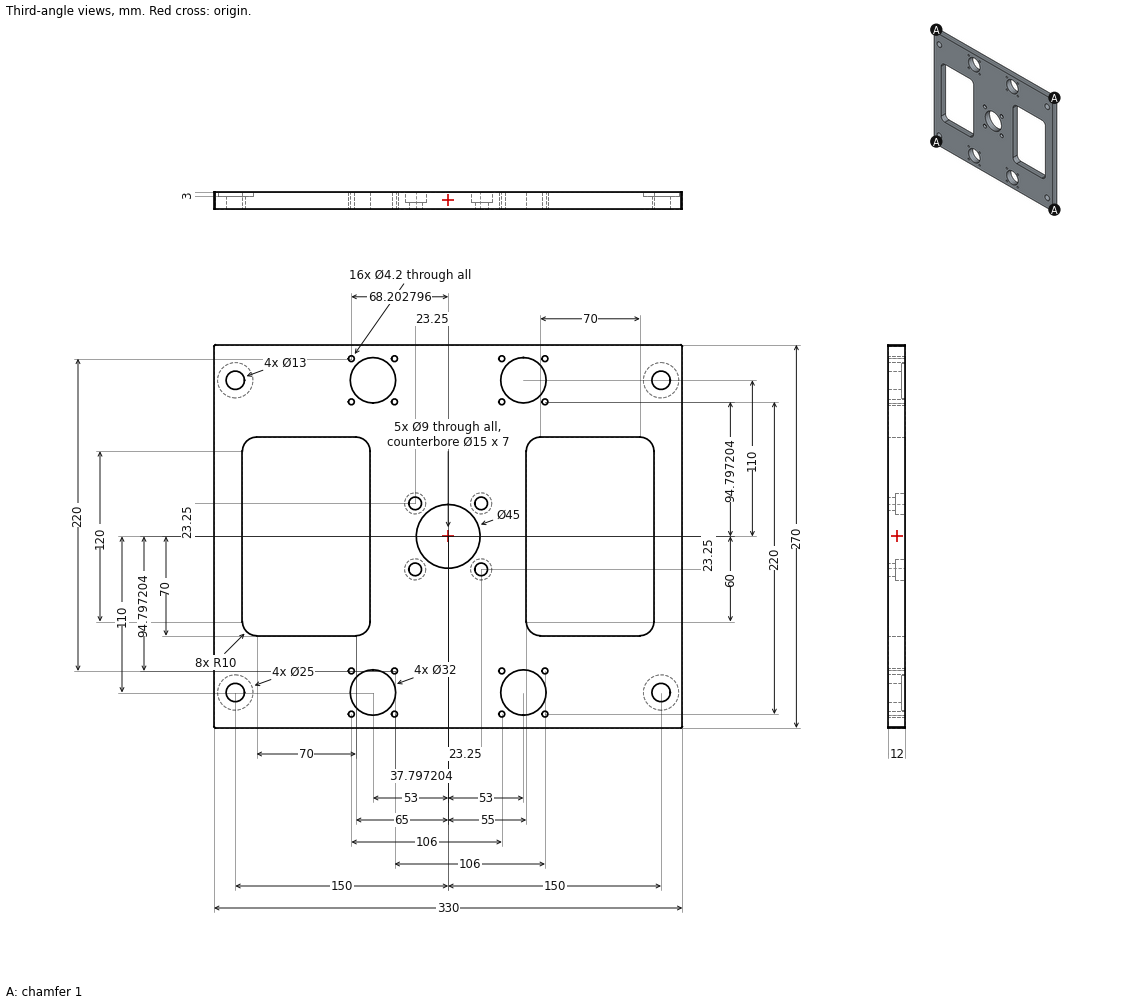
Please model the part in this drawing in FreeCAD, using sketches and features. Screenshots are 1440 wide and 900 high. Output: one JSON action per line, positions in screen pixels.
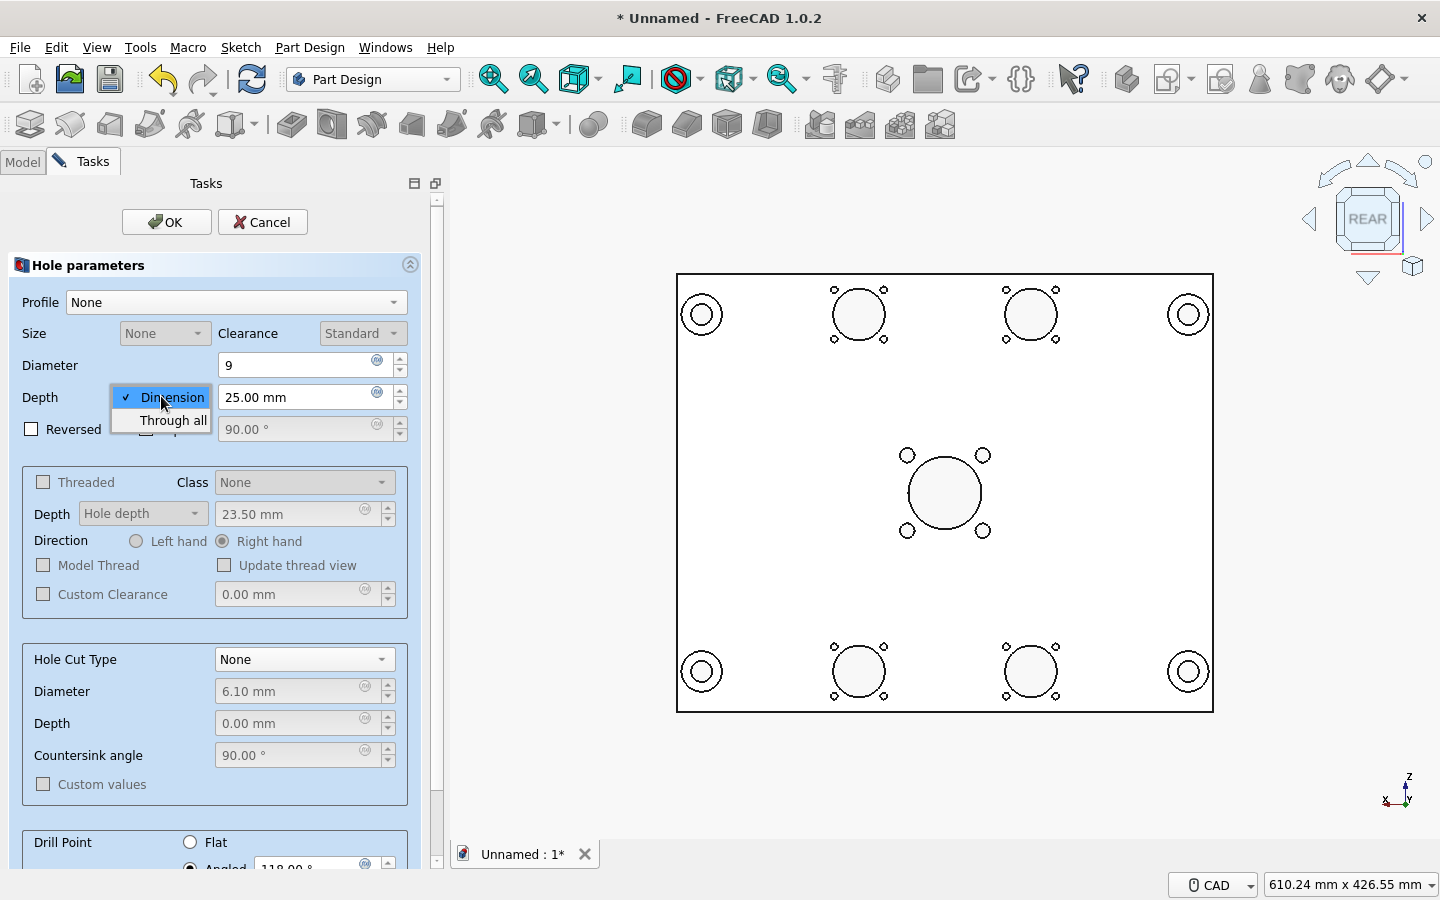
{"action": "left_click", "coordinate": [160, 420]}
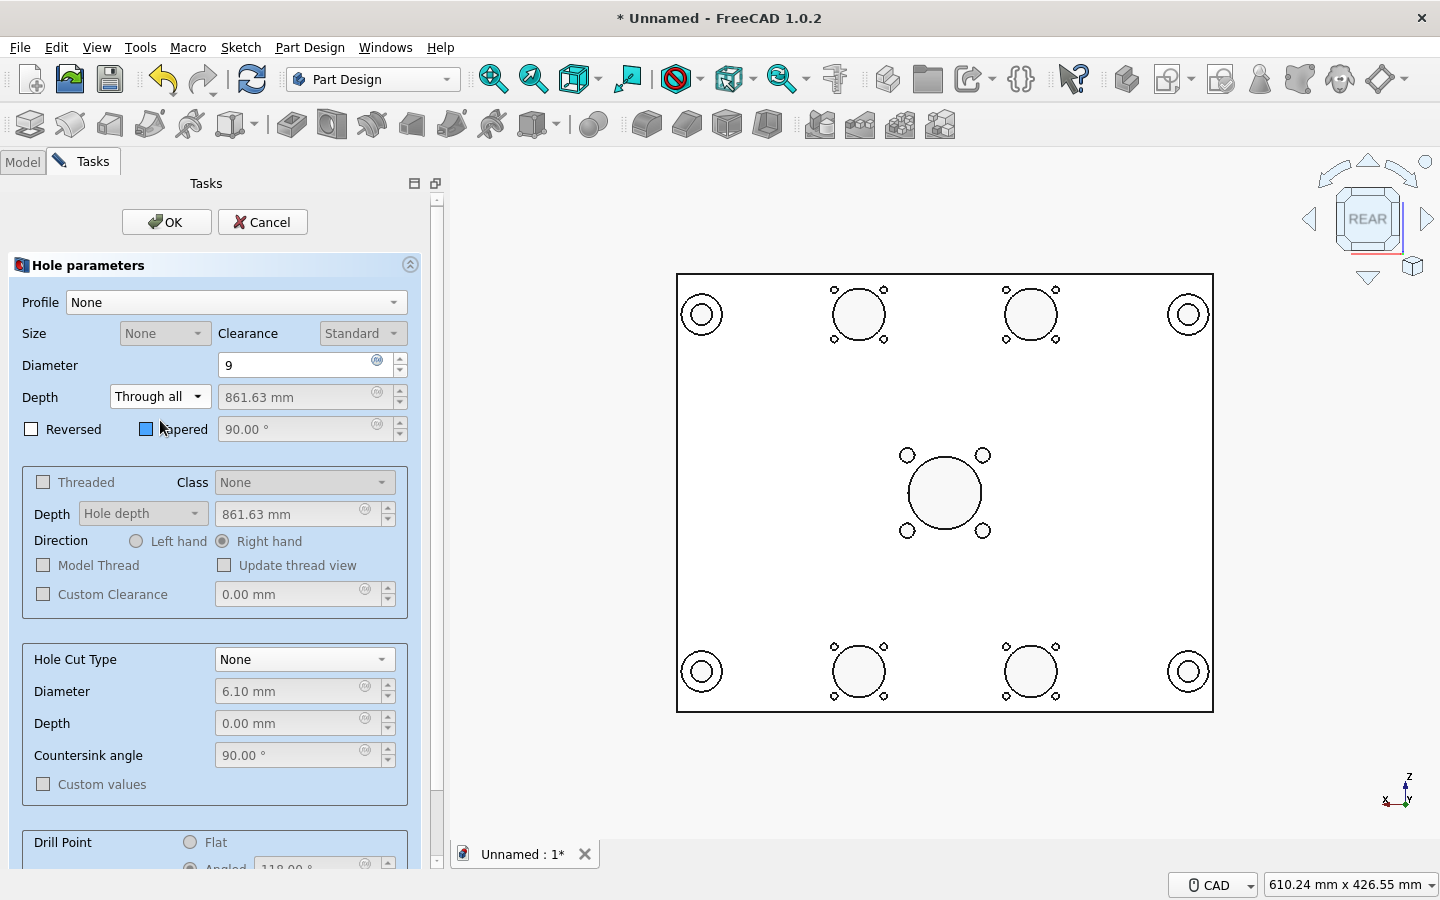
{"action": "left_click", "coordinate": [306, 660]}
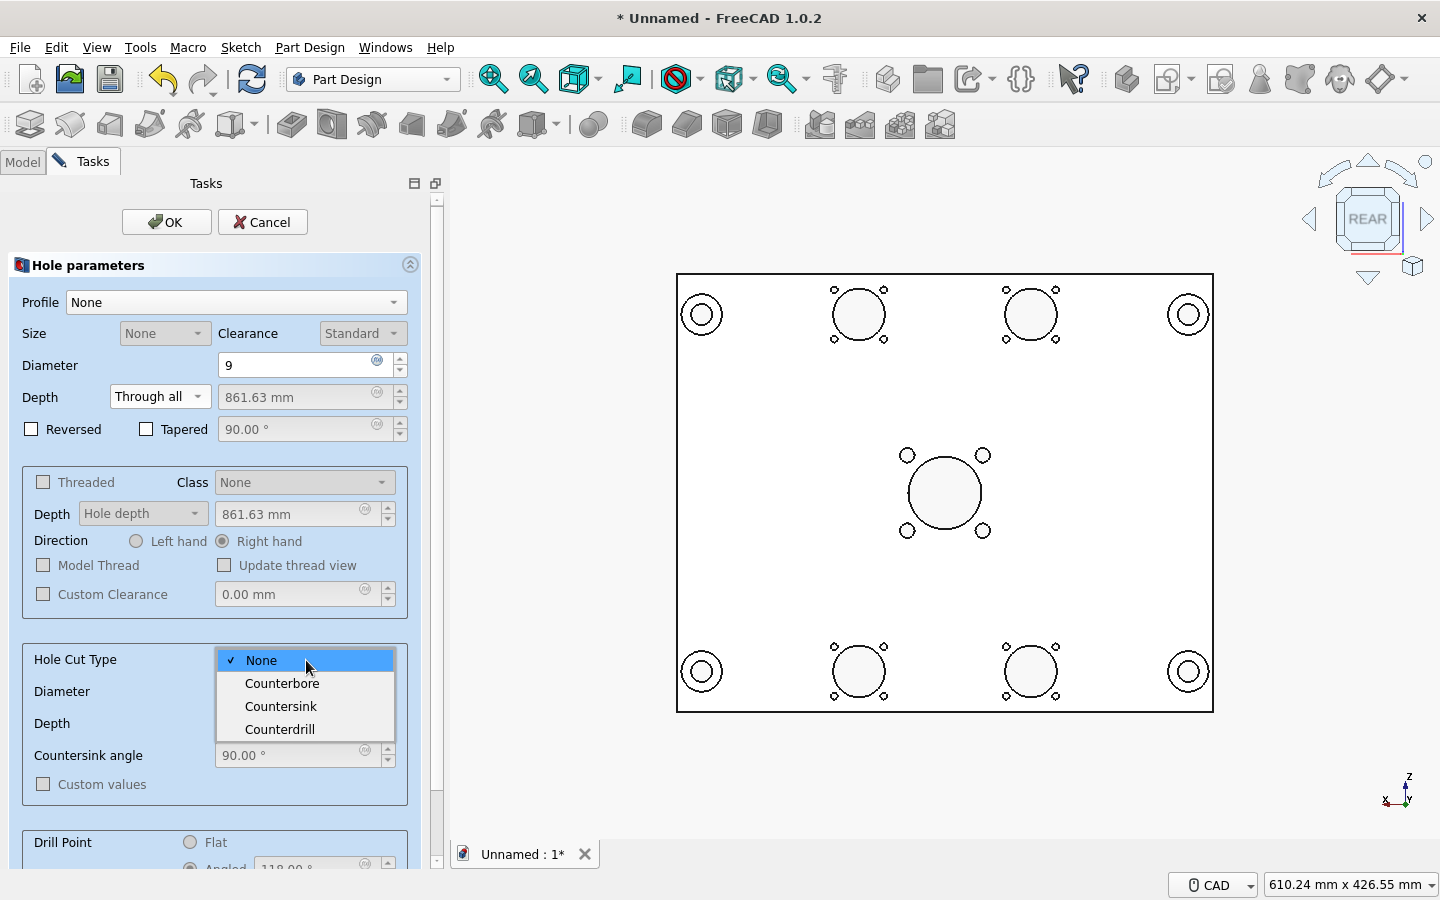
{"action": "left_click", "coordinate": [304, 684]}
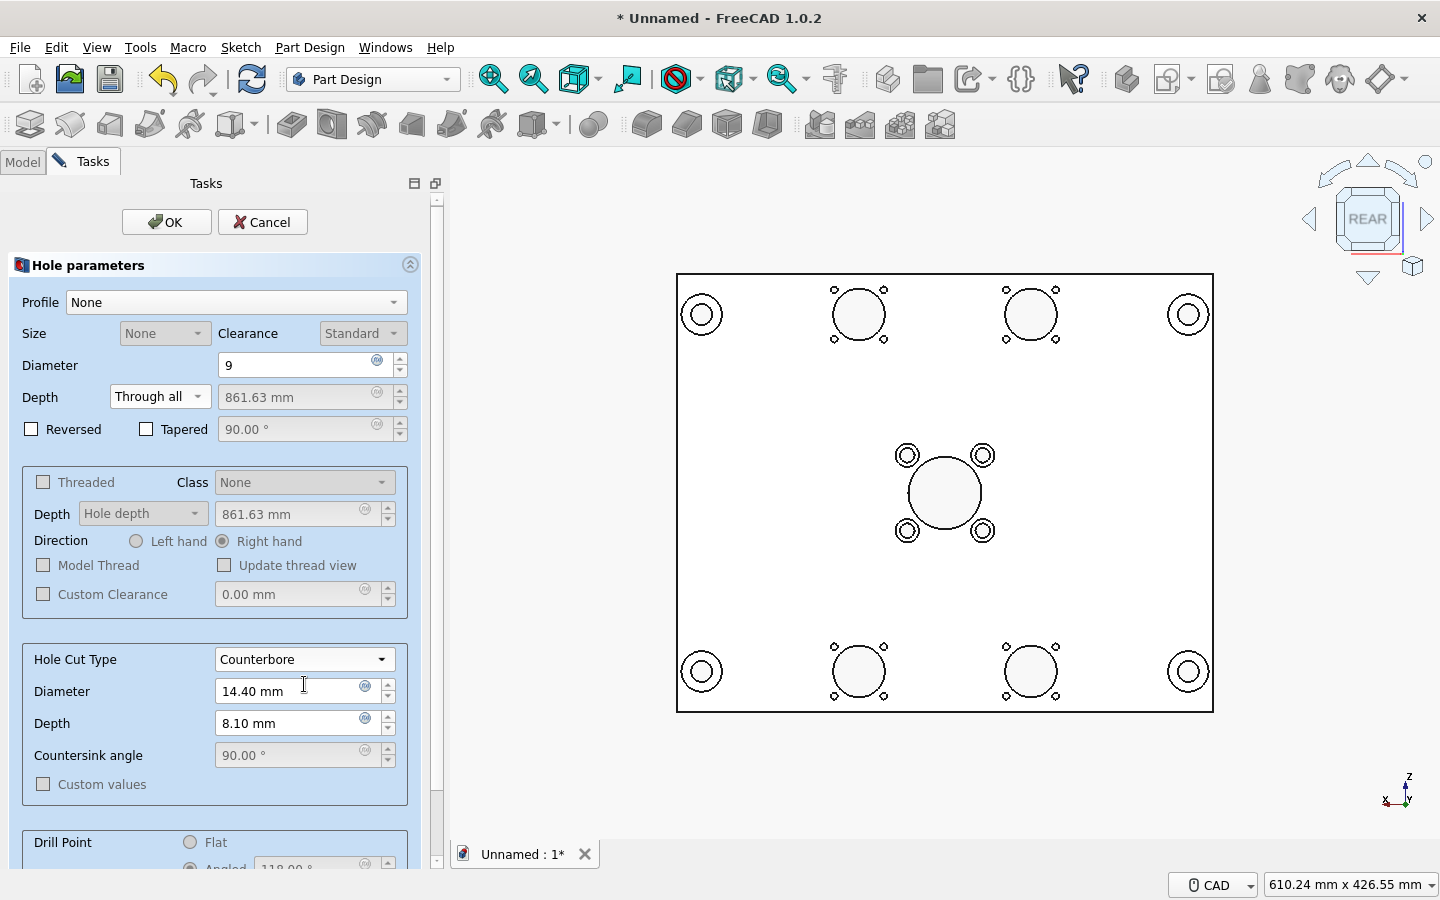
{"action": "triple_click", "coordinate": [298, 691]}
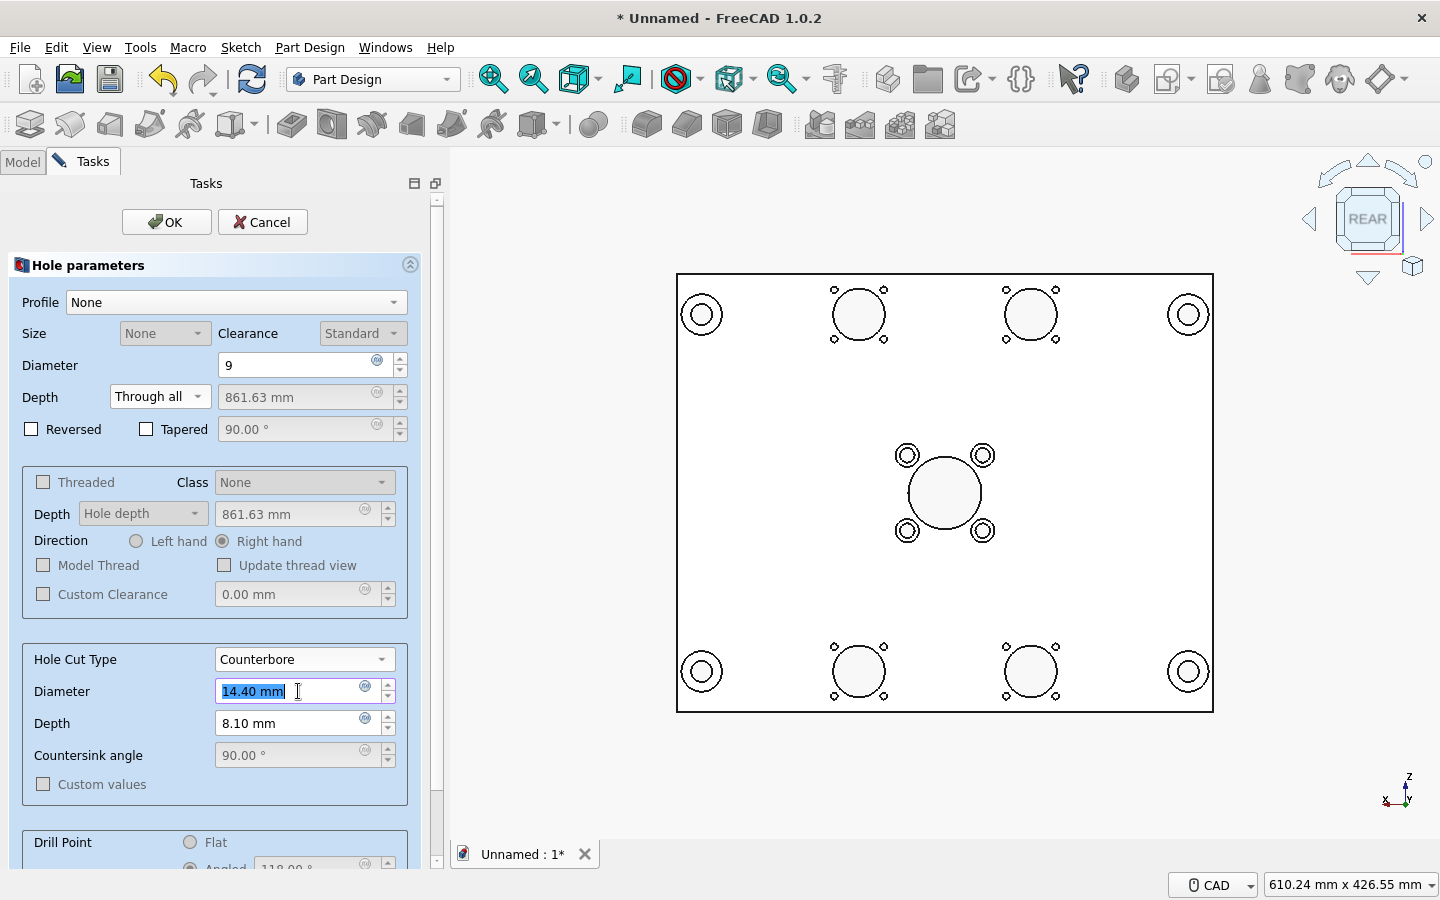
{"action": "type", "text": "15"}
{"action": "key", "text": "Tab"}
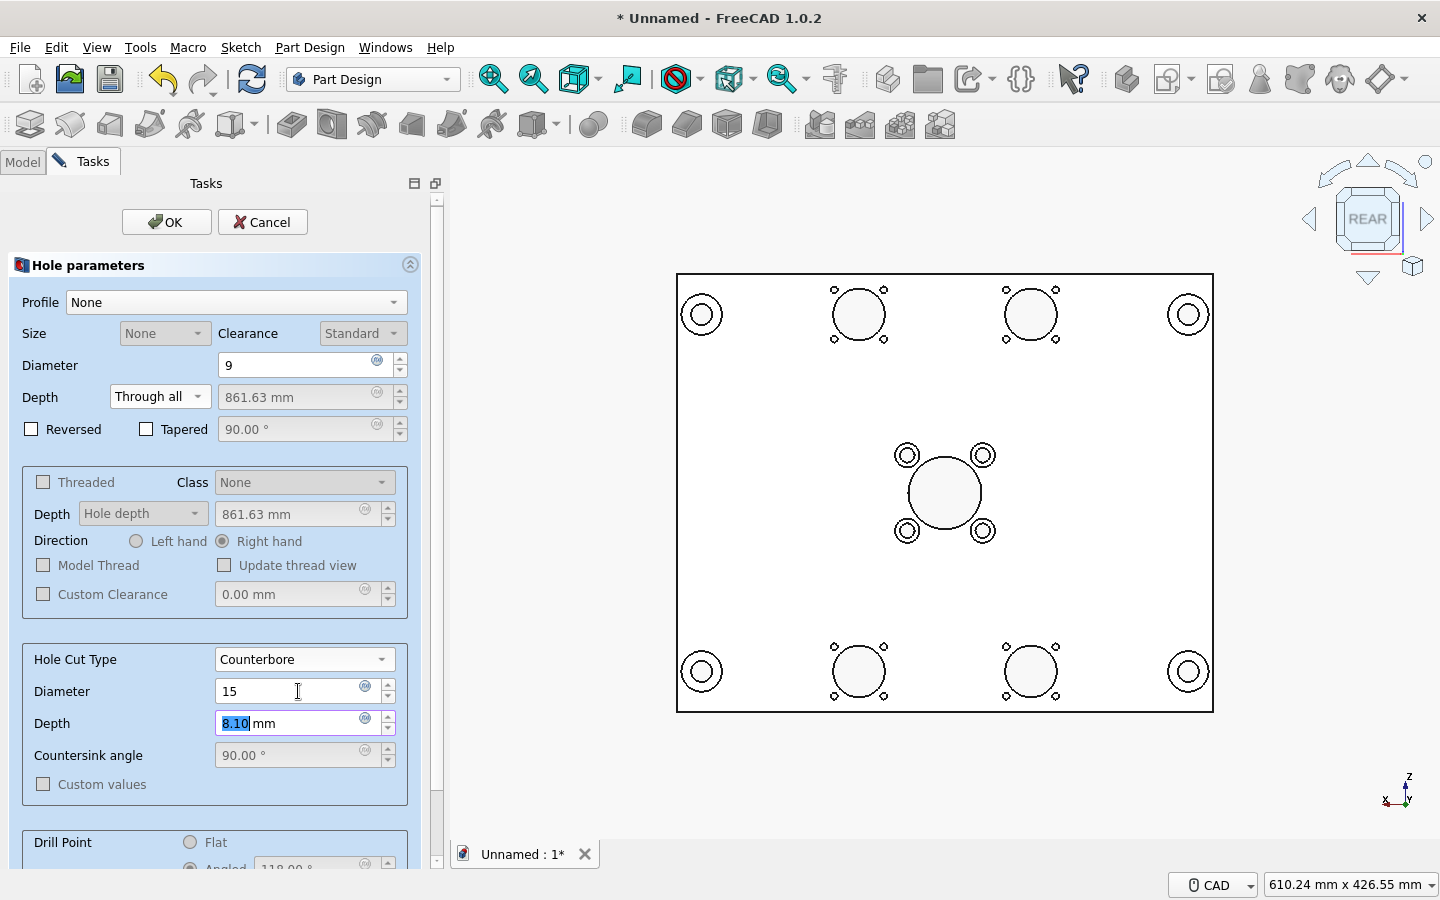
{"action": "type", "text": "7"}
{"action": "key", "text": "Tab"}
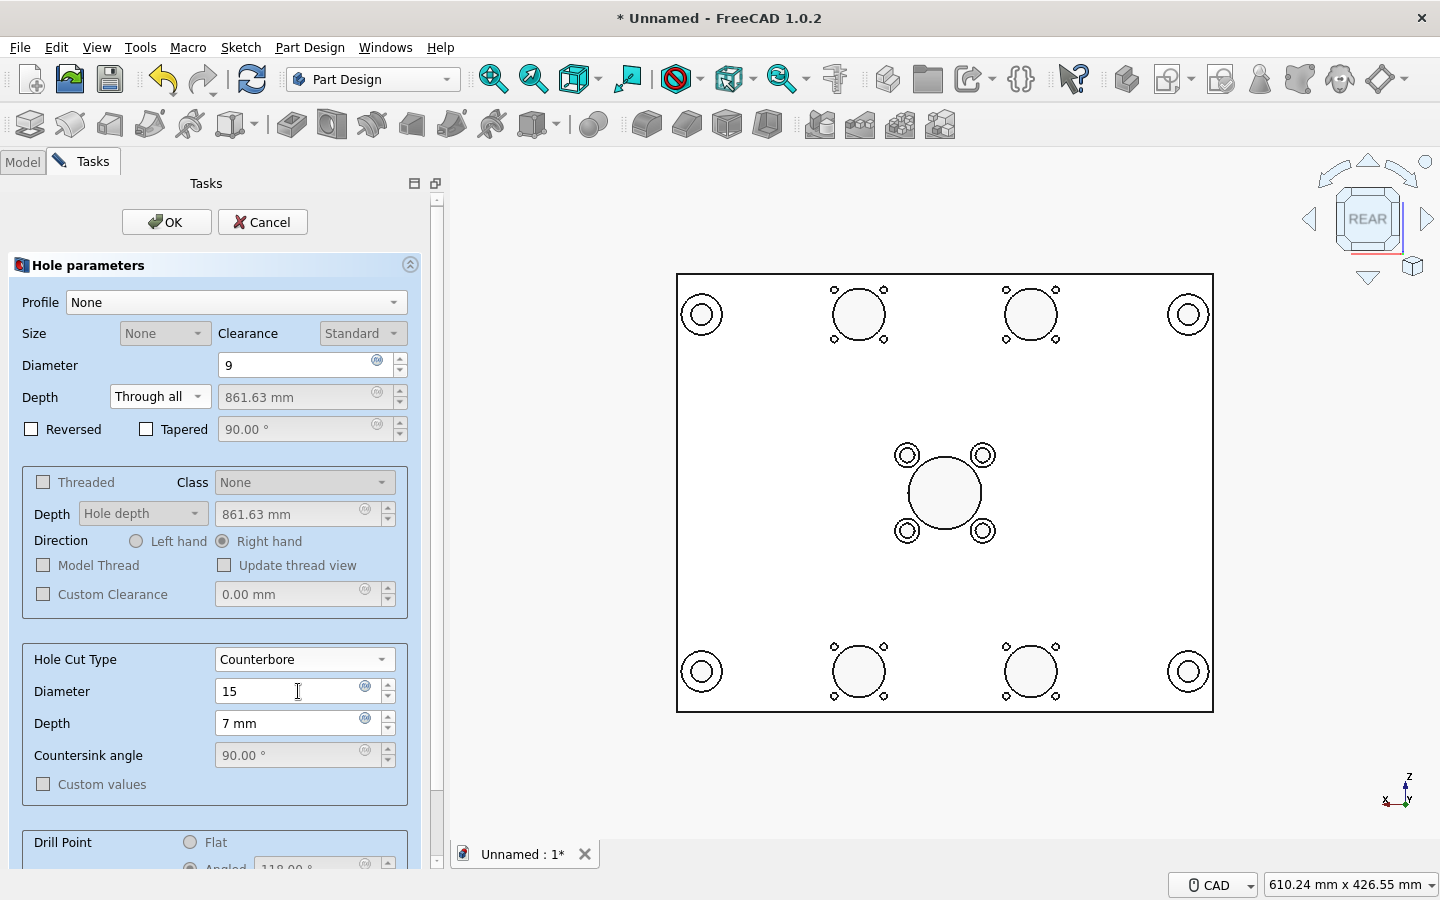
{"action": "left_click", "coordinate": [167, 222]}